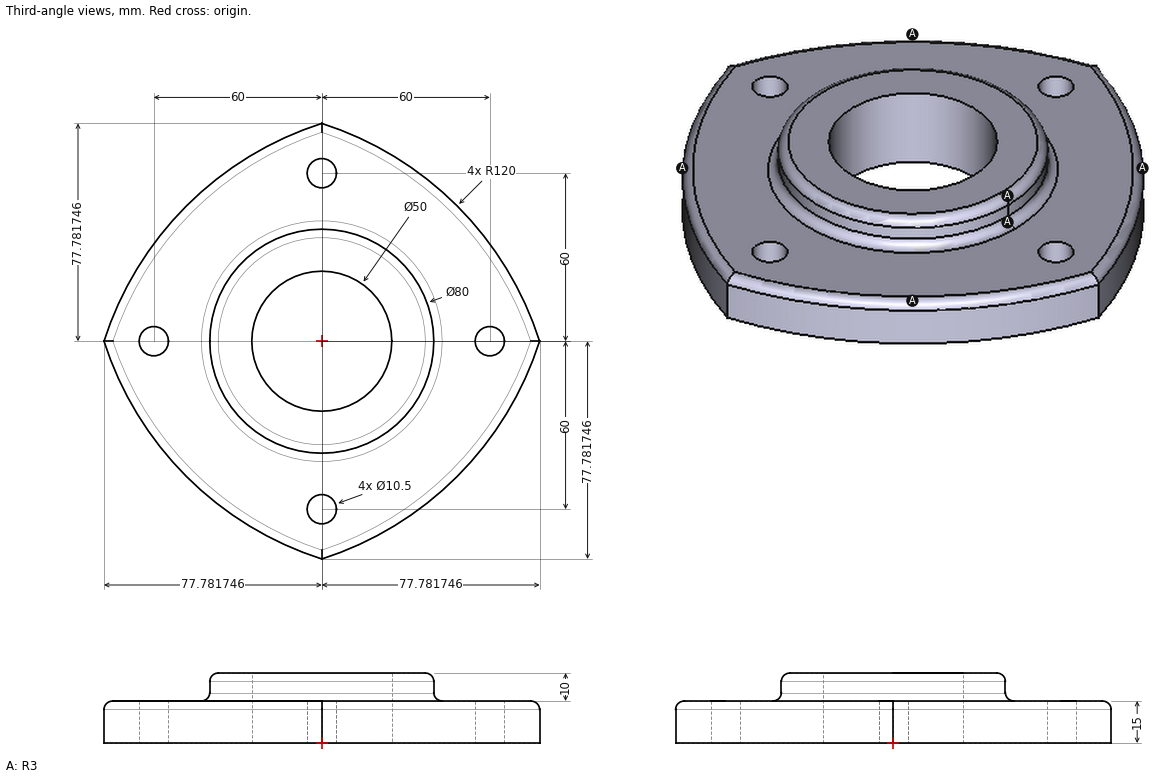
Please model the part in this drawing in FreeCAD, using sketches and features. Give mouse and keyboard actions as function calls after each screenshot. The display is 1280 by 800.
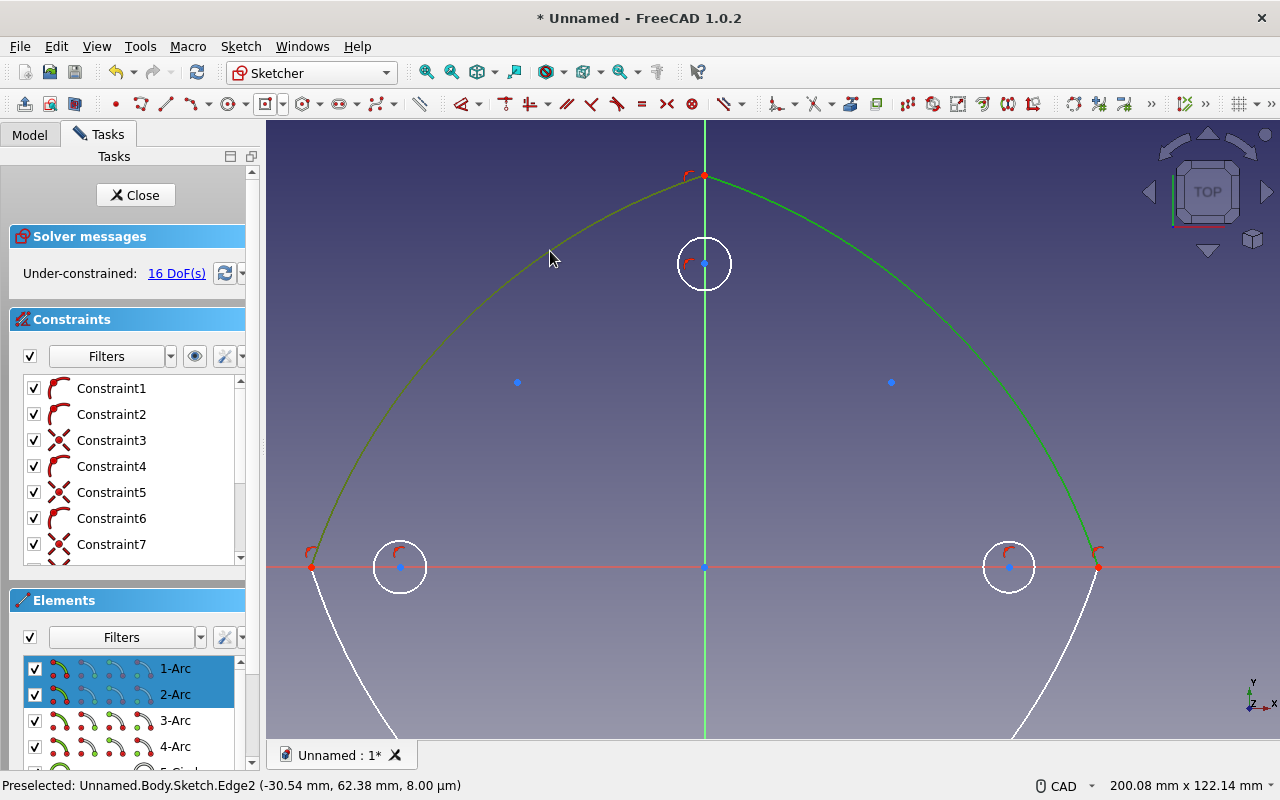
click(356, 674)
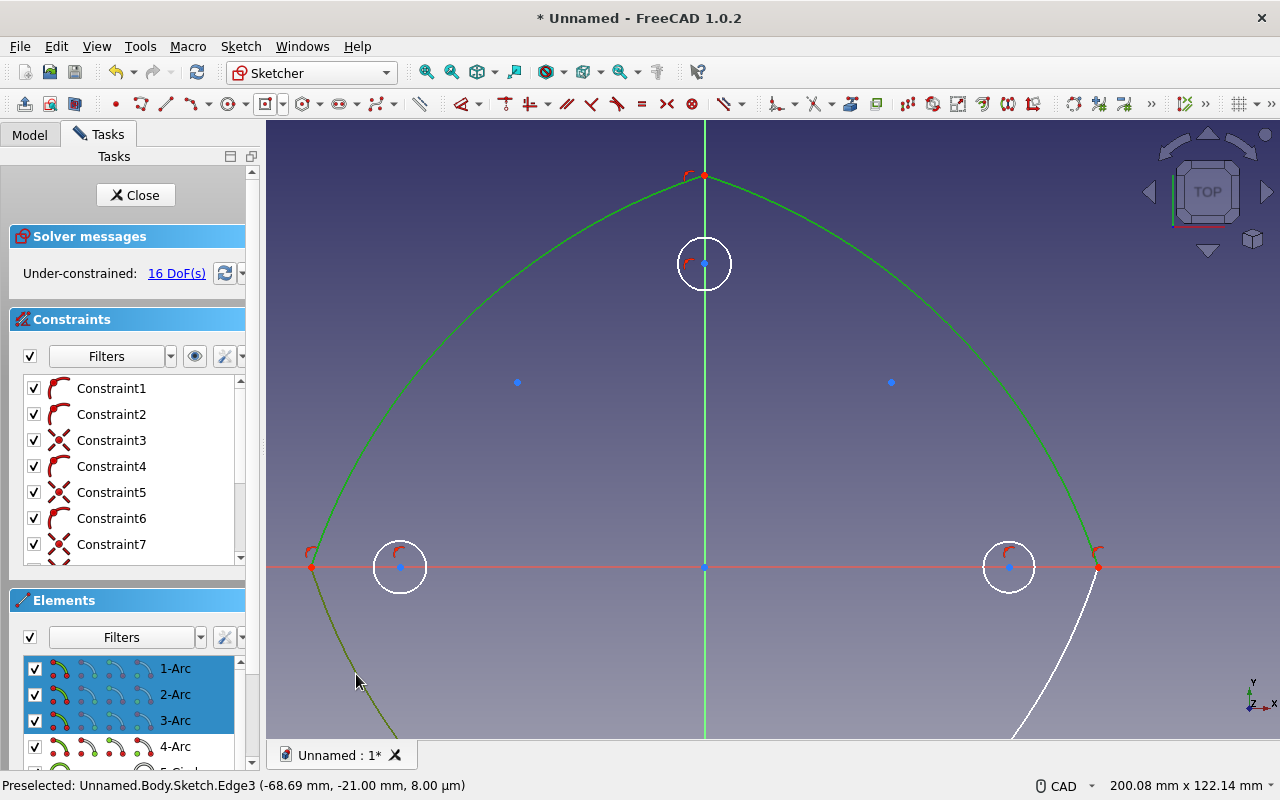
click(1053, 674)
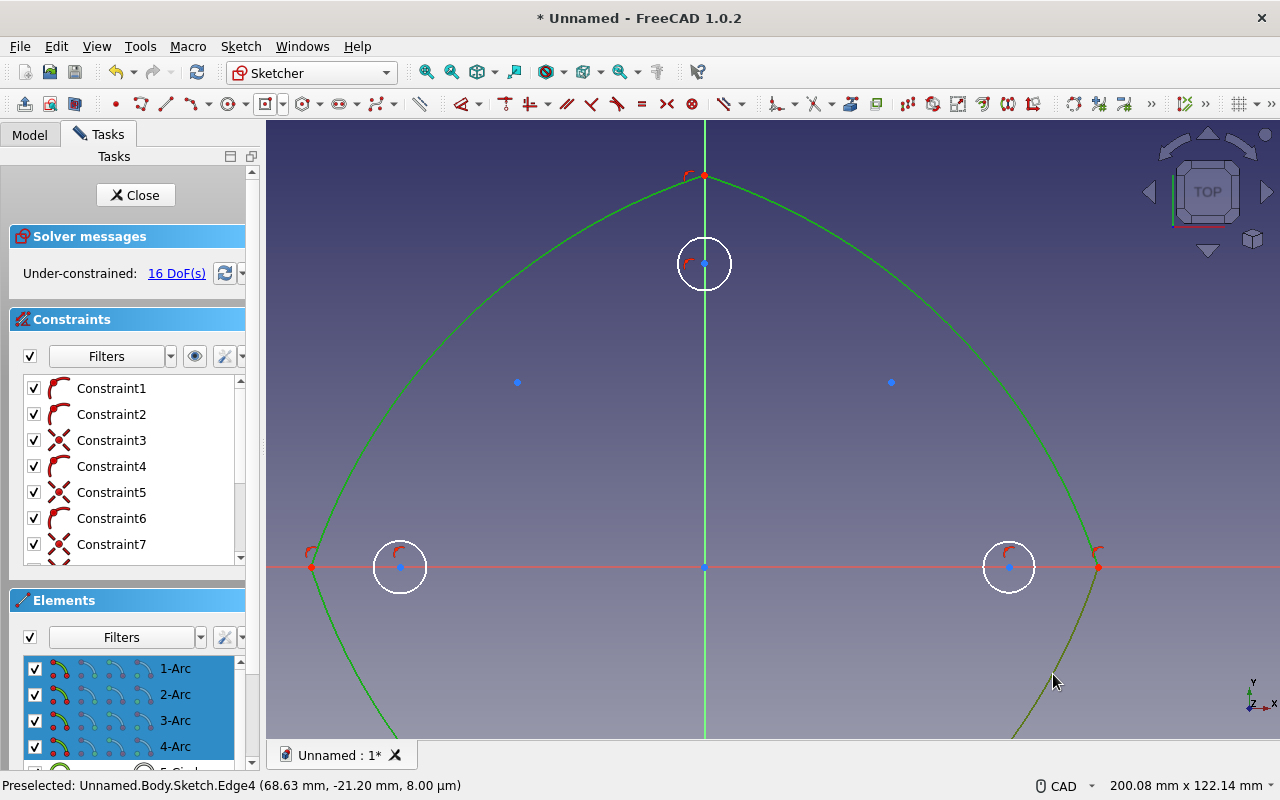
key(e)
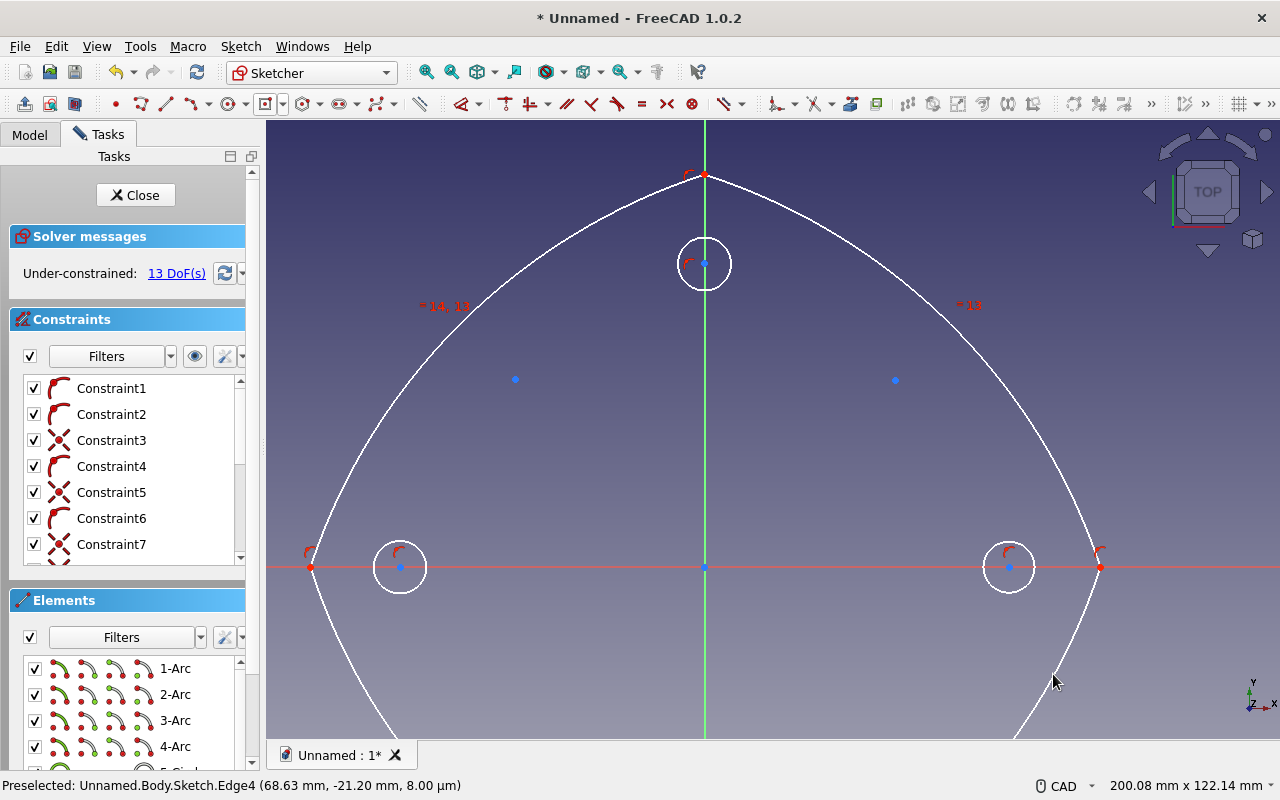
scroll(704, 262, down, 3)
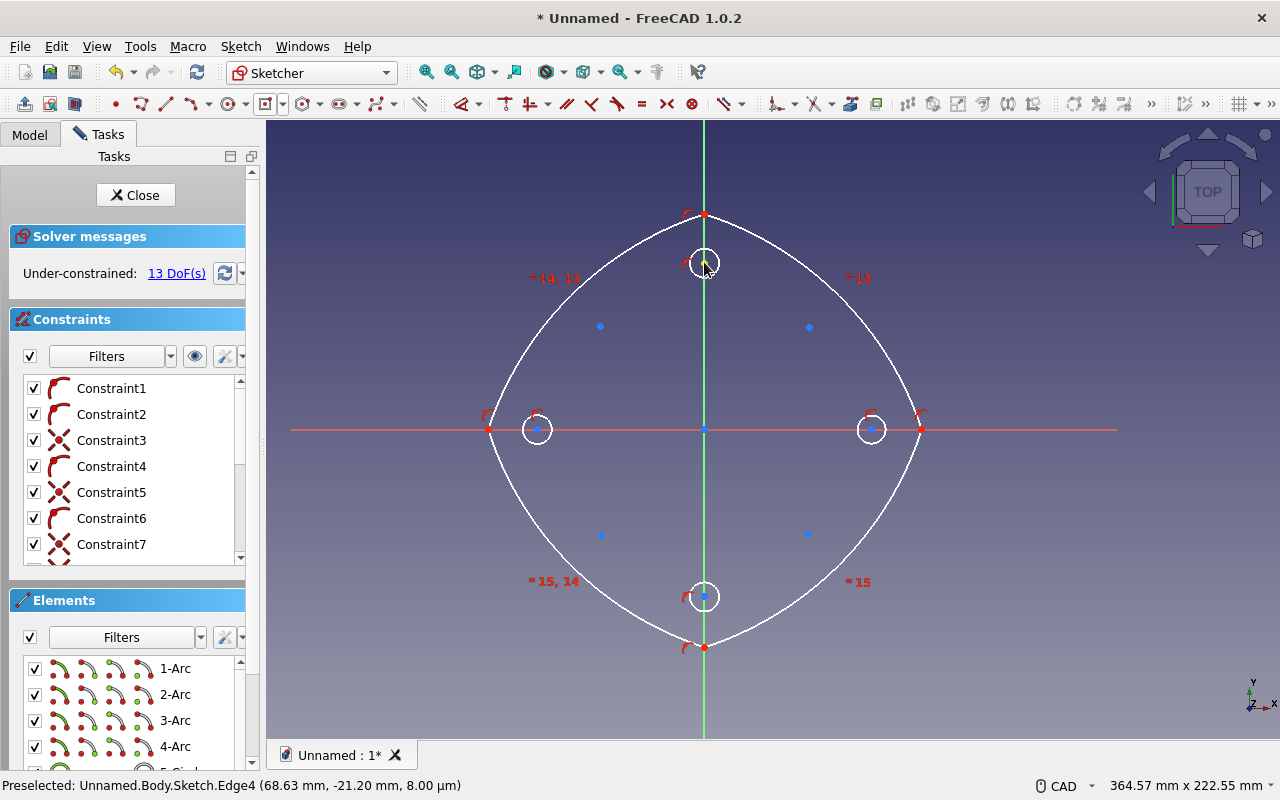
scroll(715, 587, up, 2)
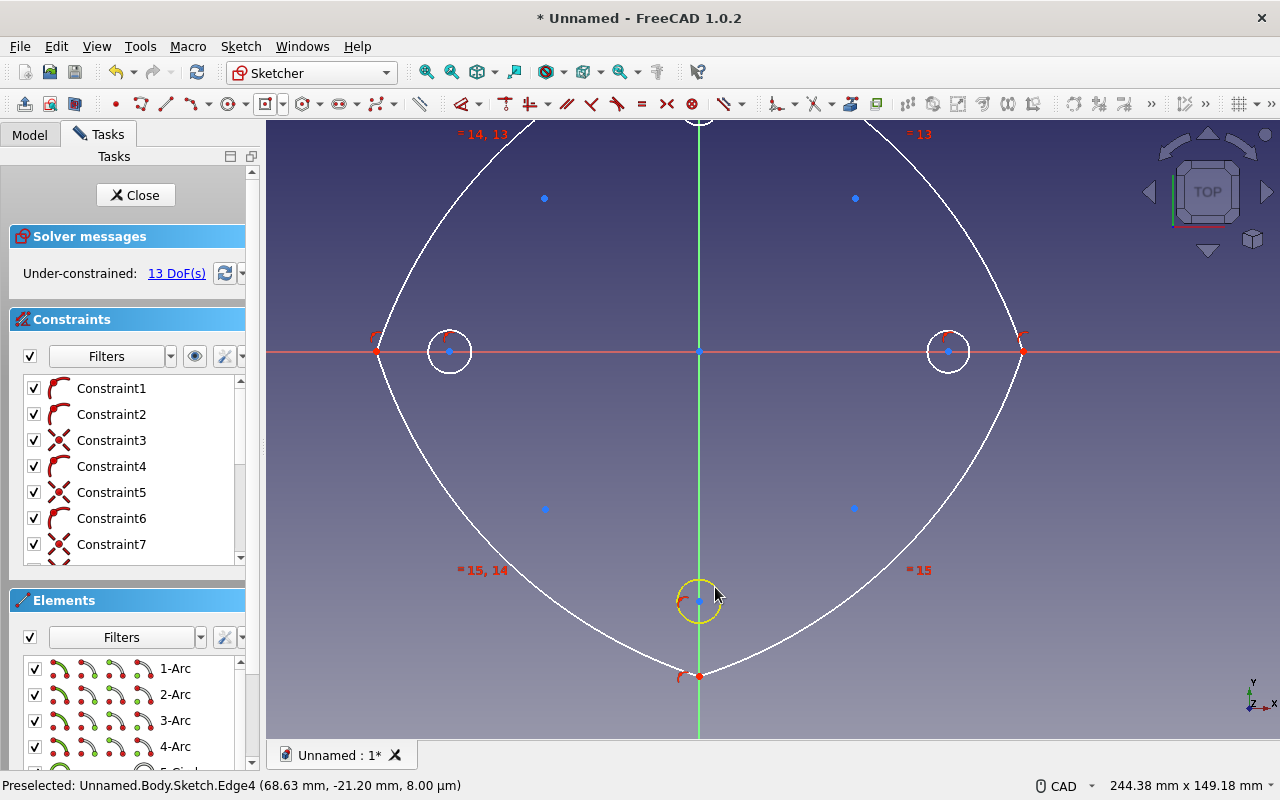
click(714, 586)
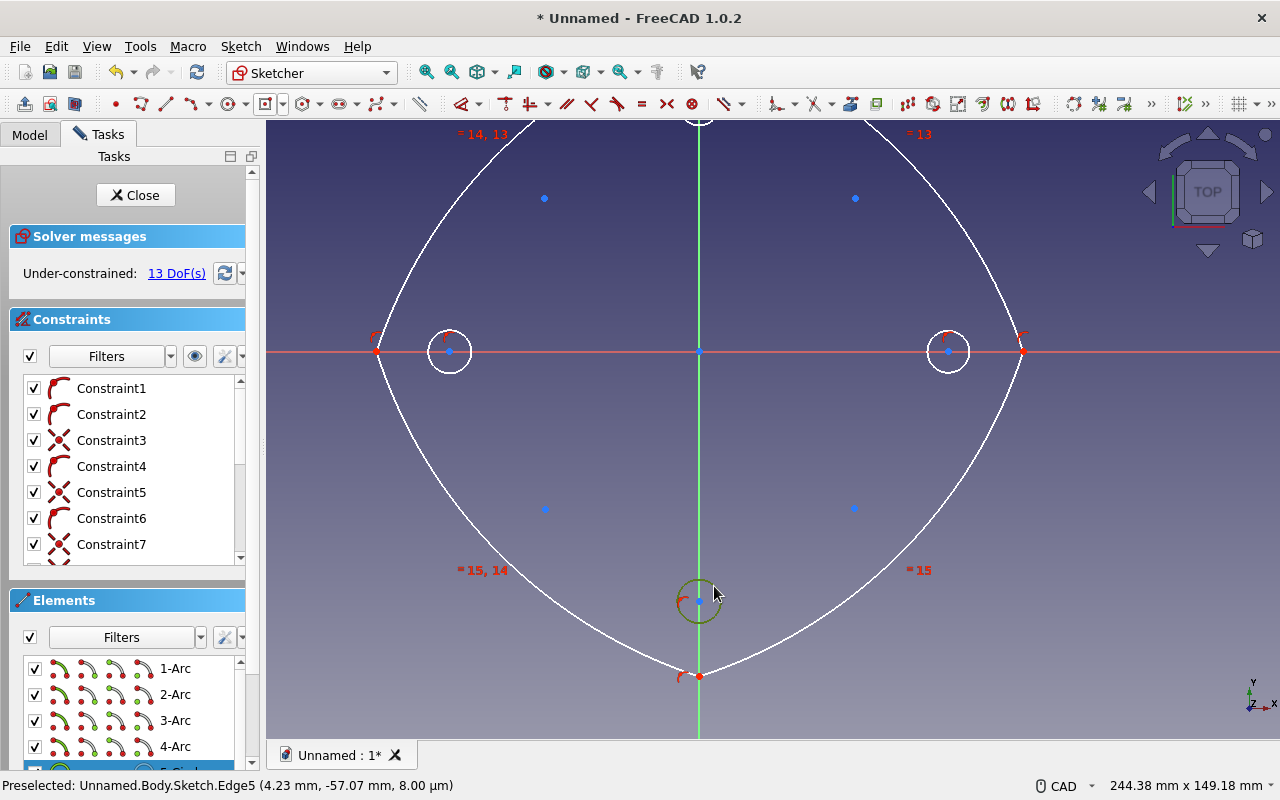
click(963, 337)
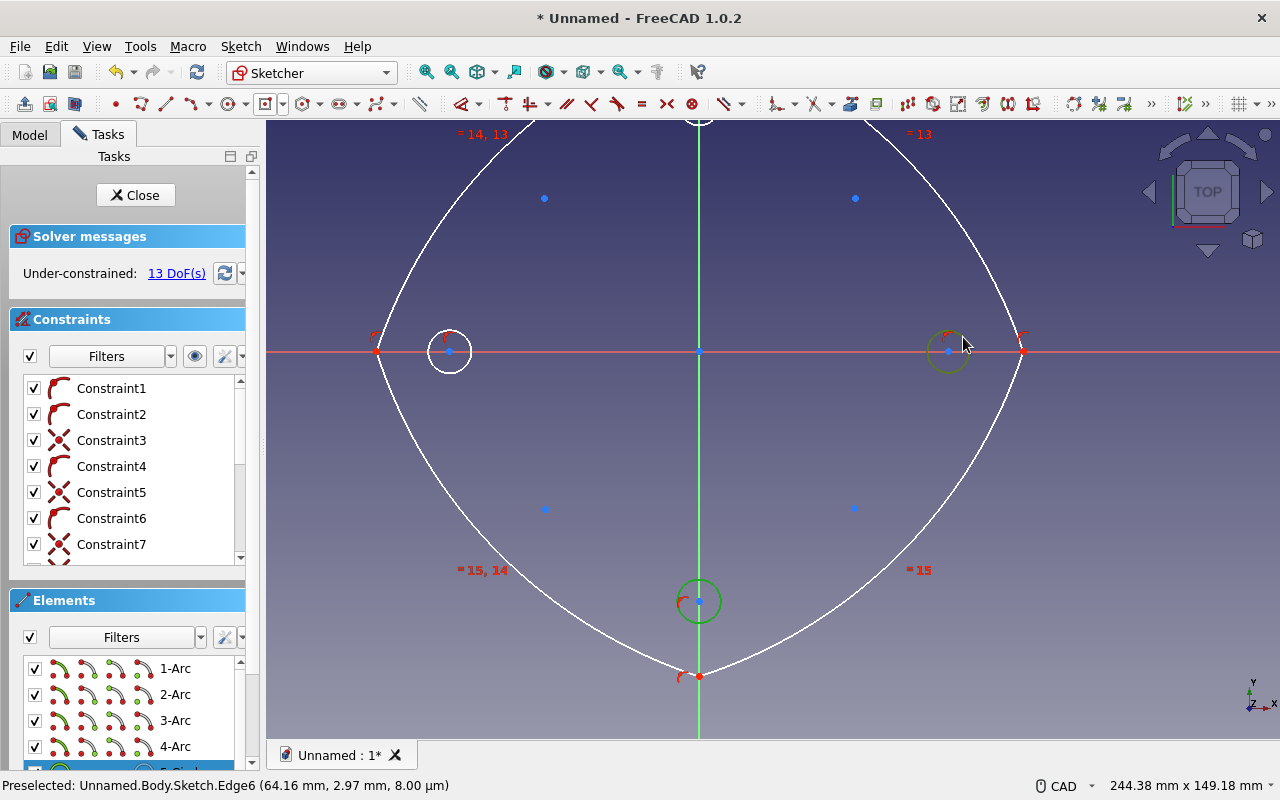
click(465, 337)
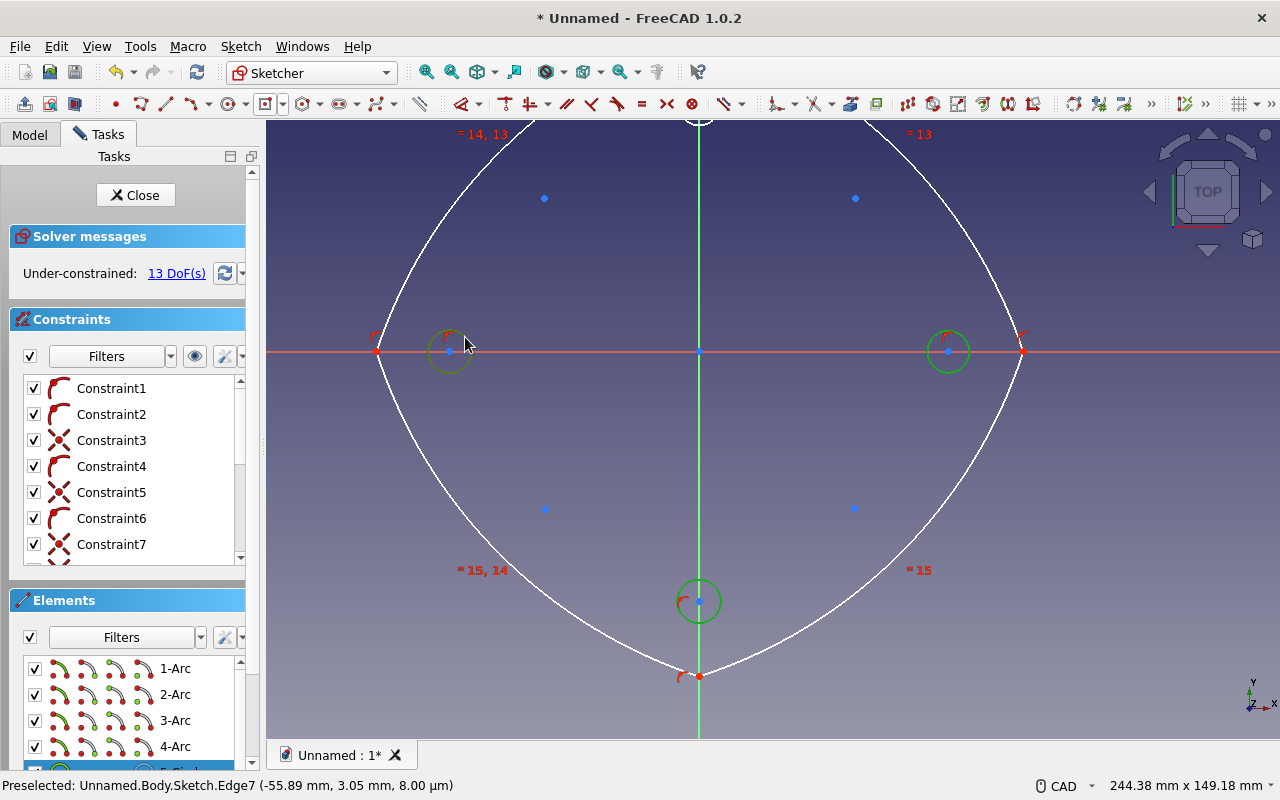
scroll(716, 587, down, 2)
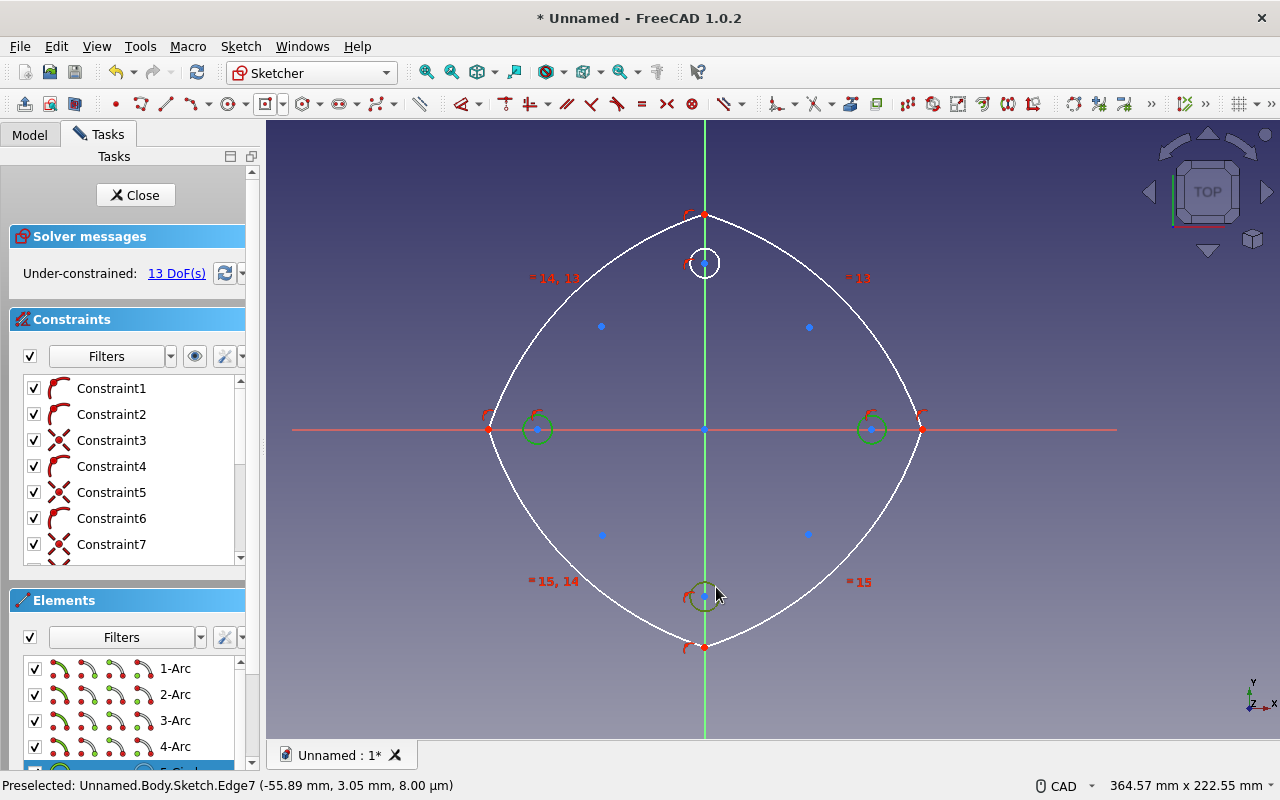
scroll(715, 253, up, 2)